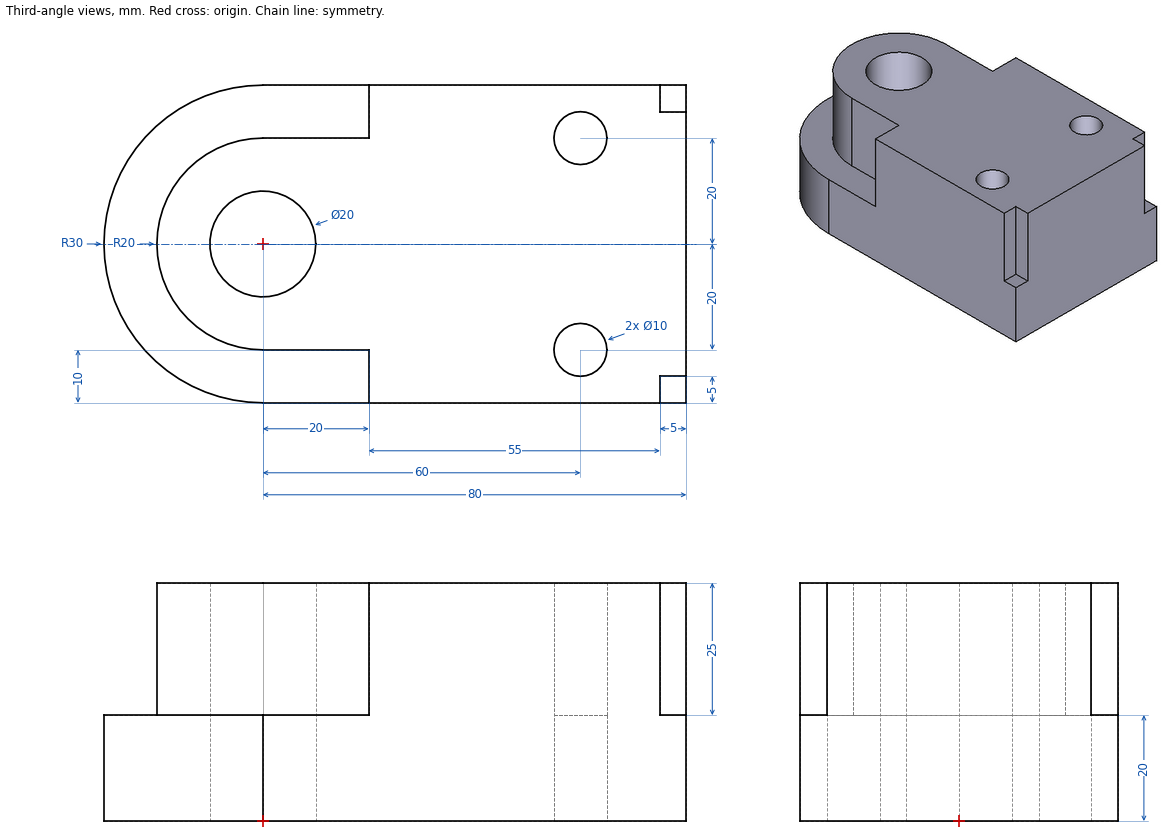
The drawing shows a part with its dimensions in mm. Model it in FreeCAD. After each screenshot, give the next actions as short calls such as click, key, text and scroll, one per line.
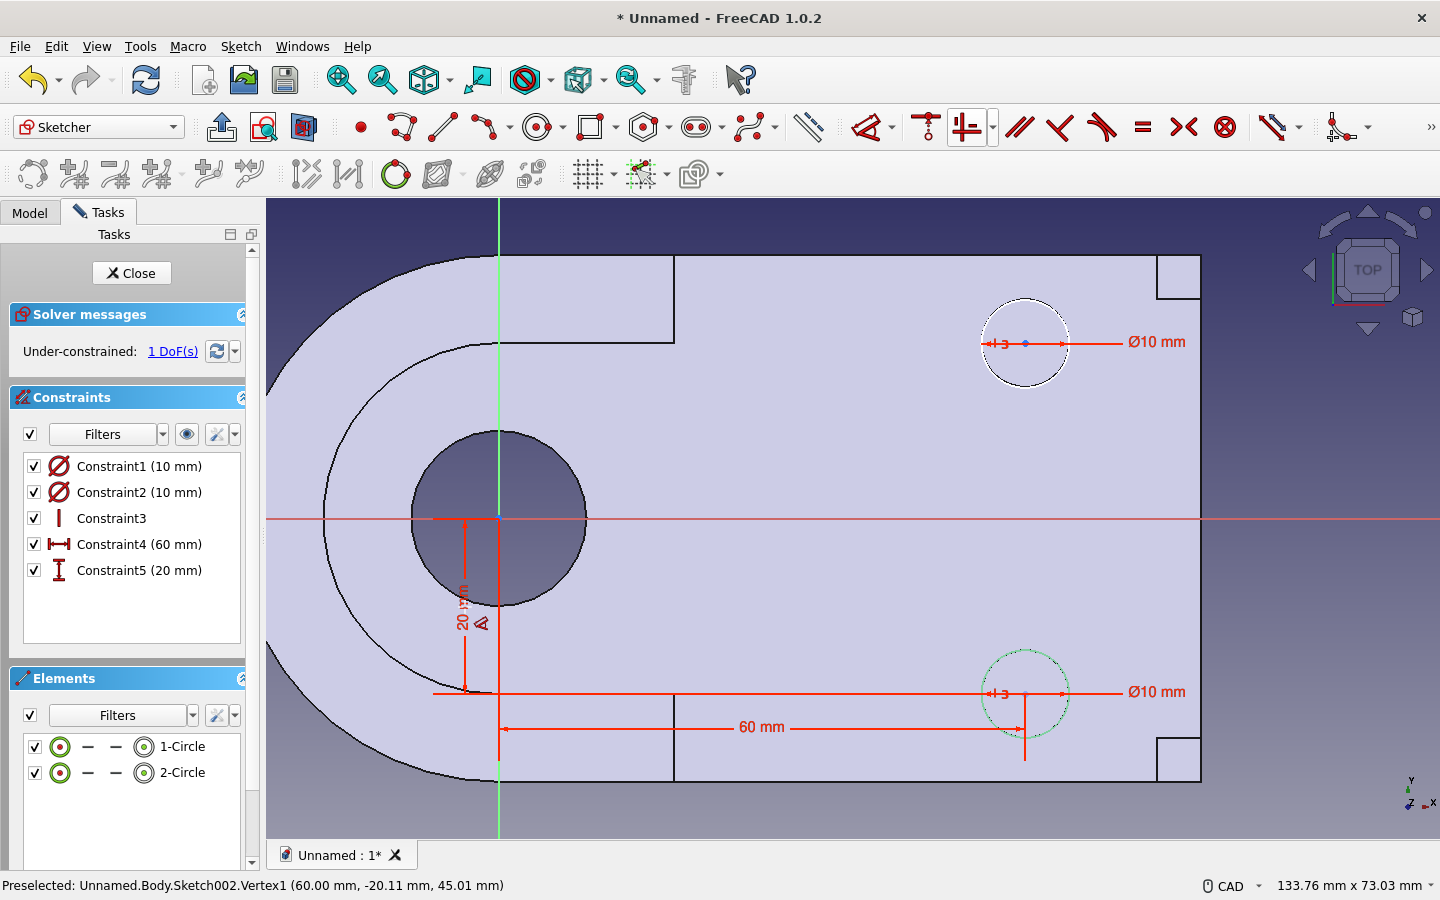
click(1025, 344)
click(465, 431)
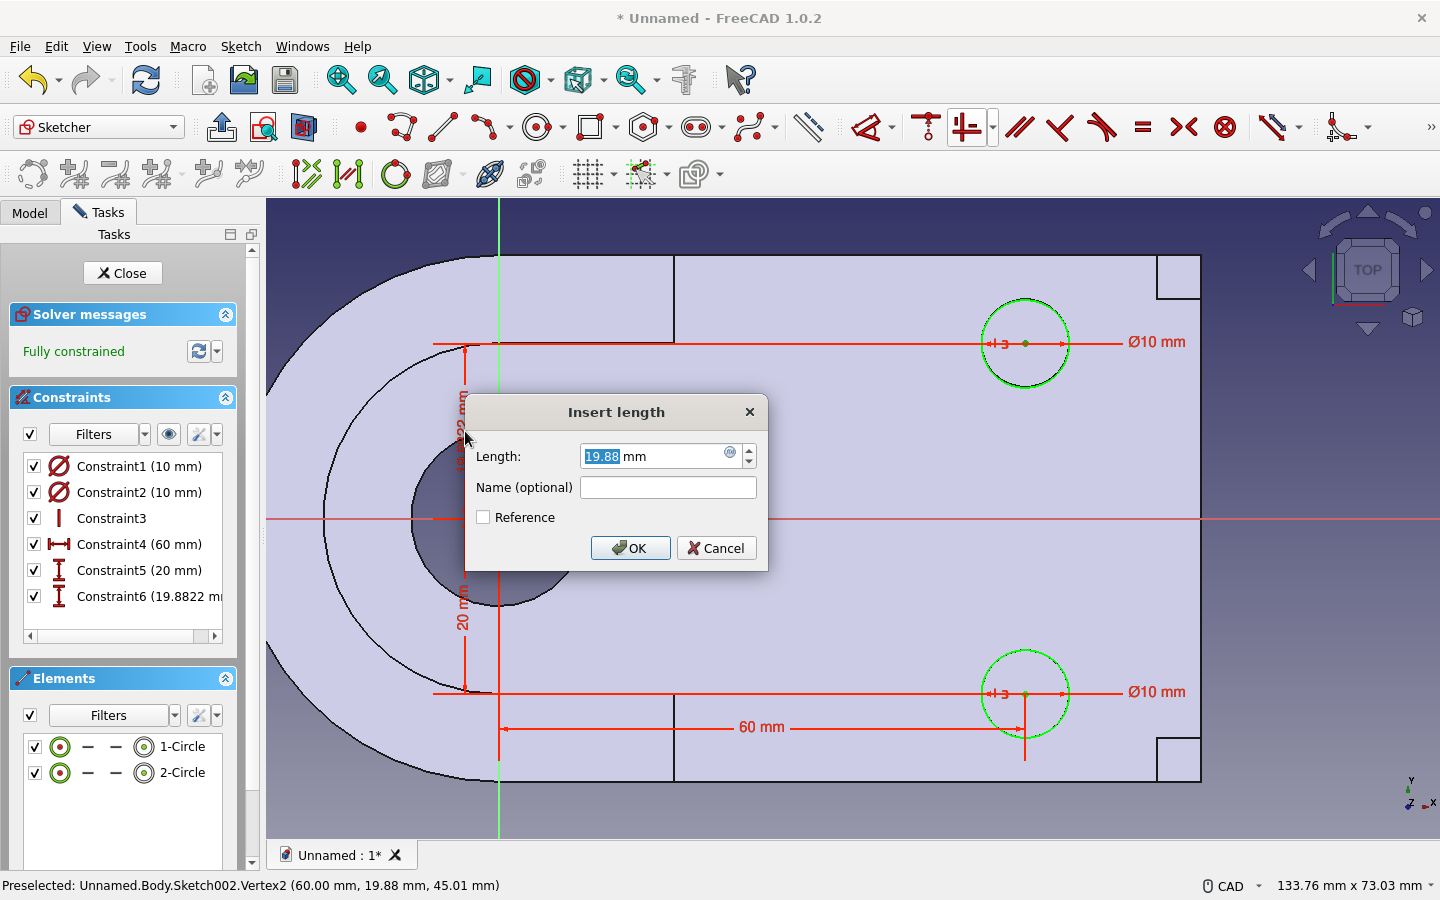
text(20)
key(Return)
key(Escape)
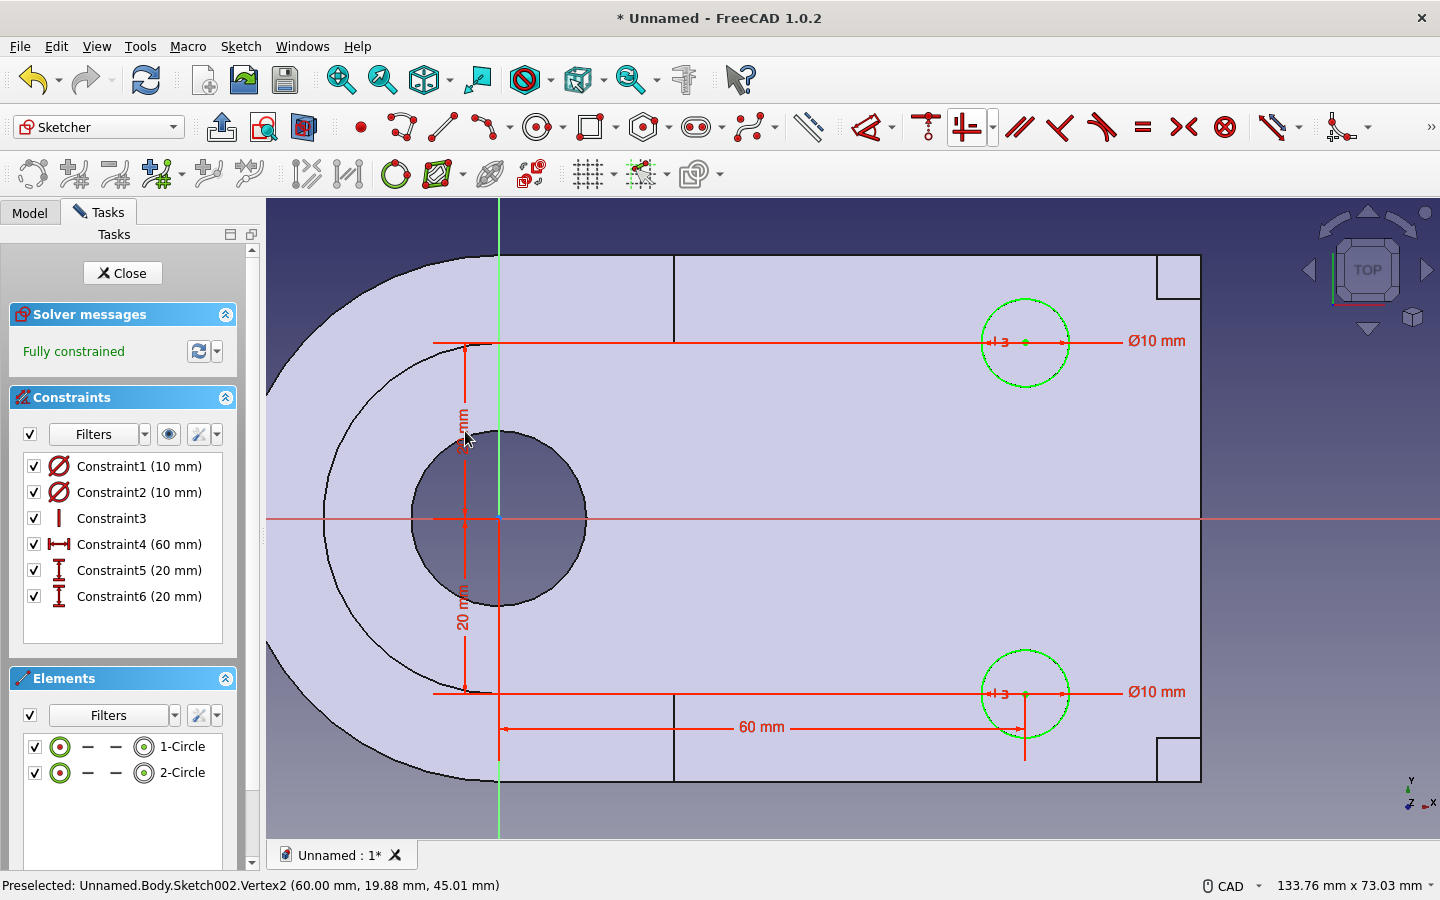
click(123, 273)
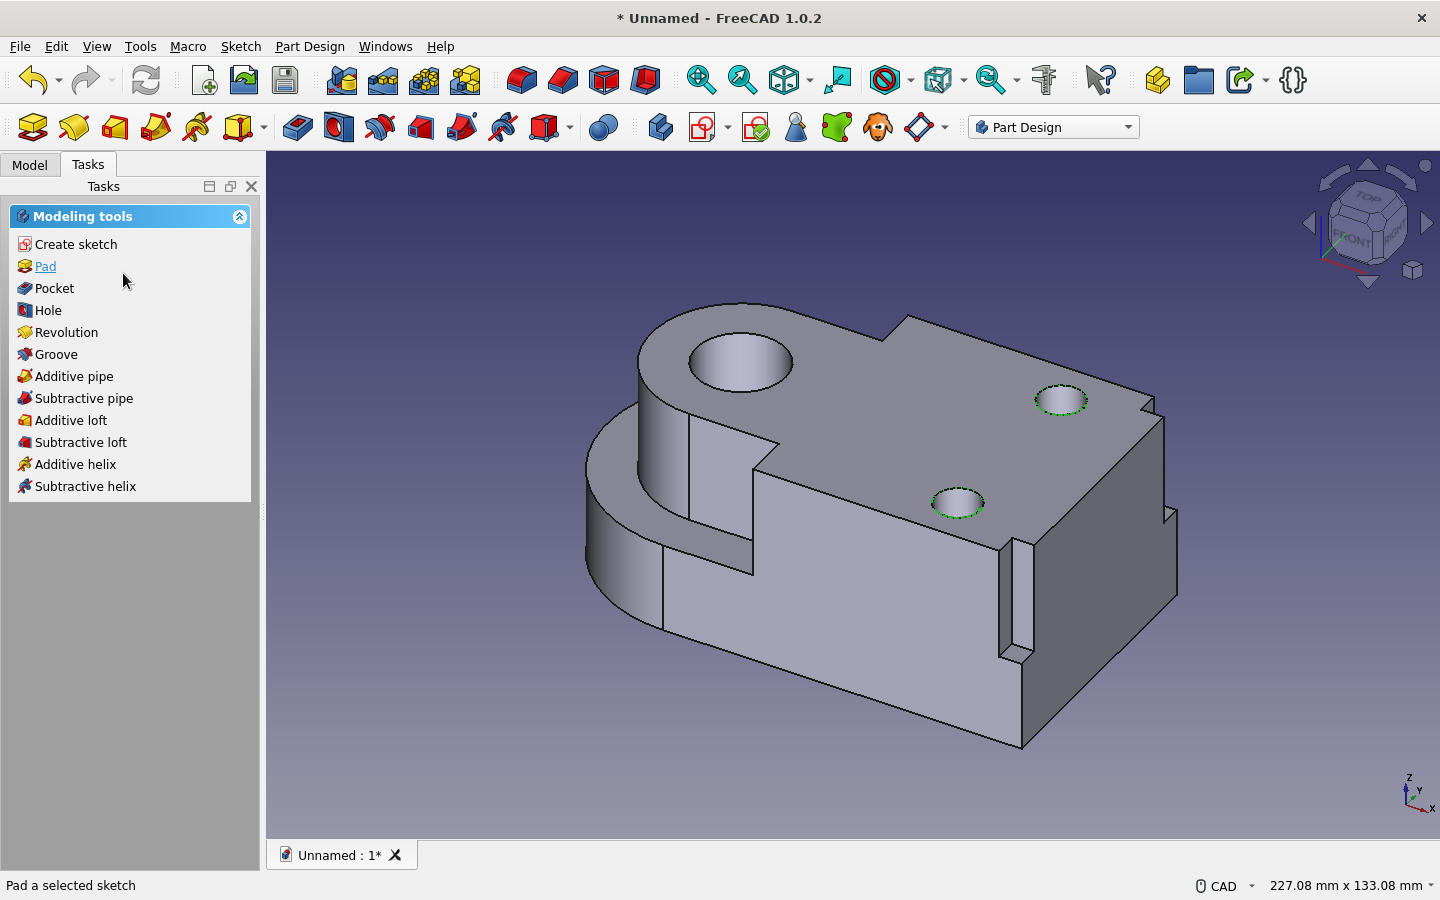
click(298, 128)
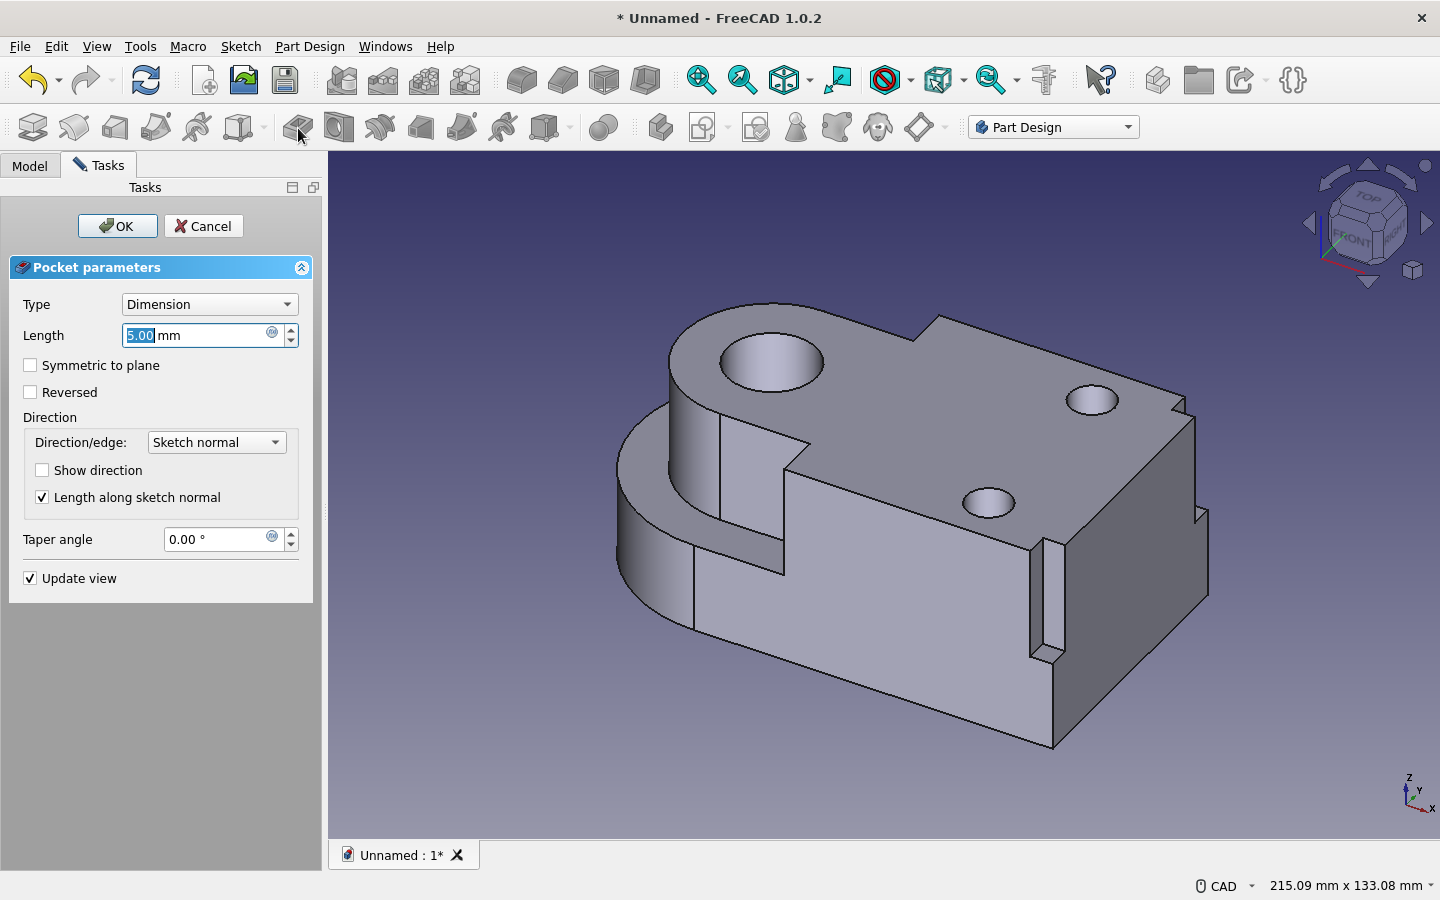
click(210, 304)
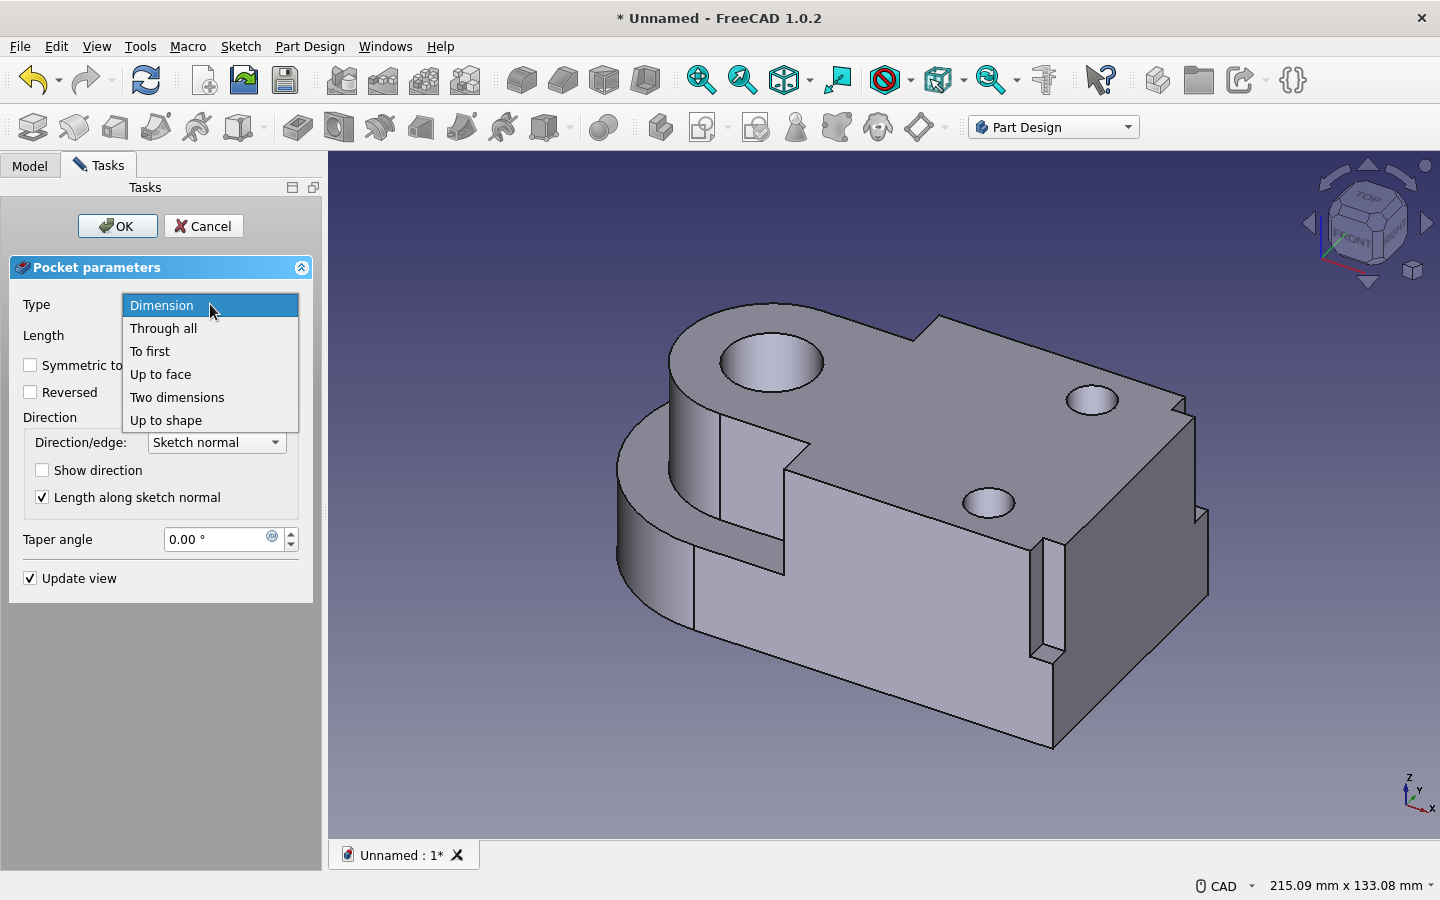
click(208, 328)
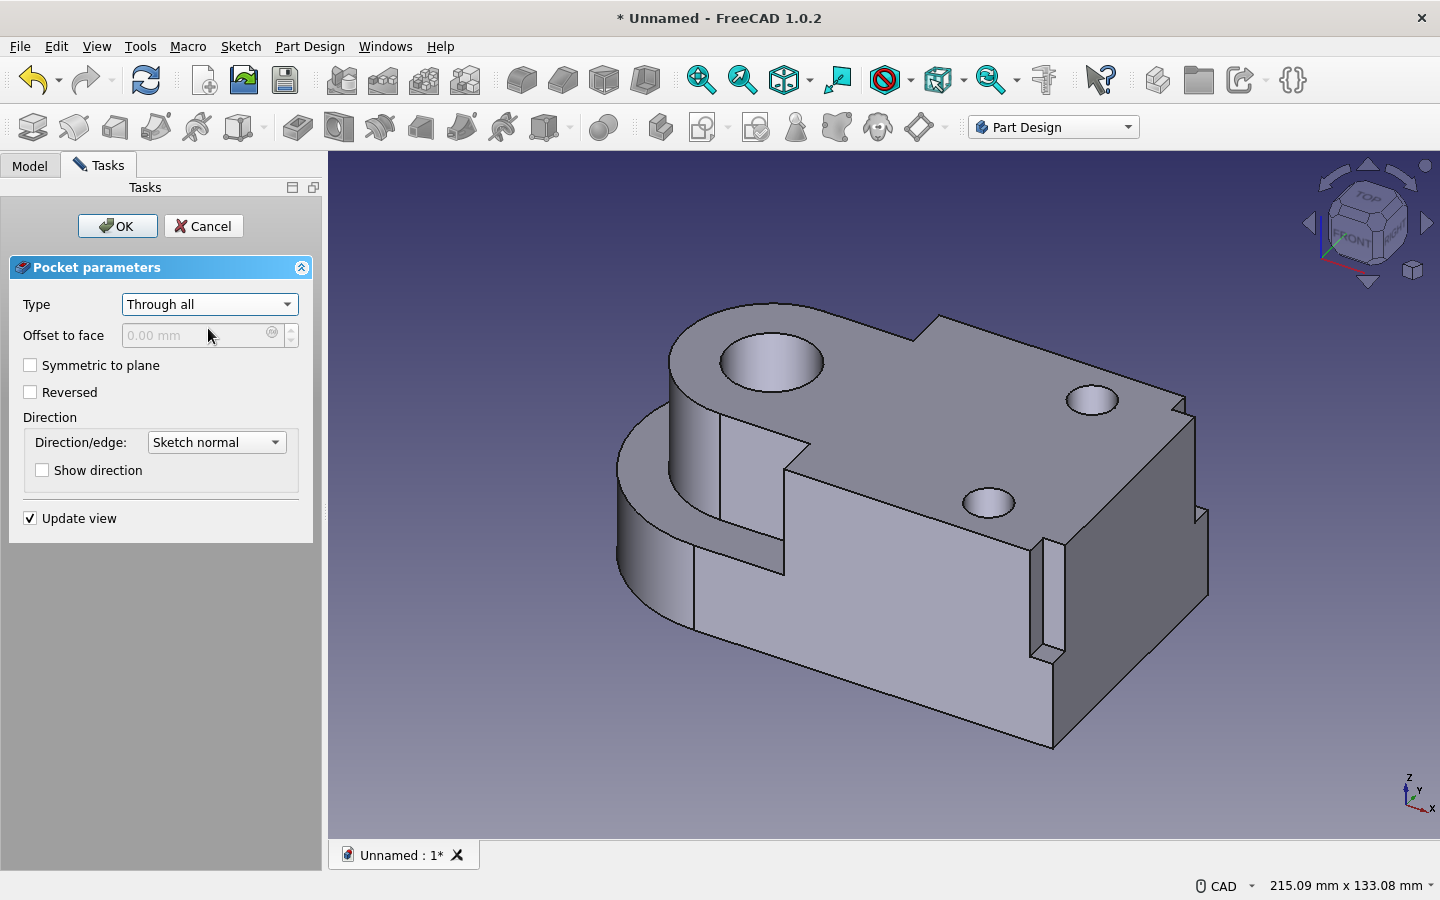
click(118, 226)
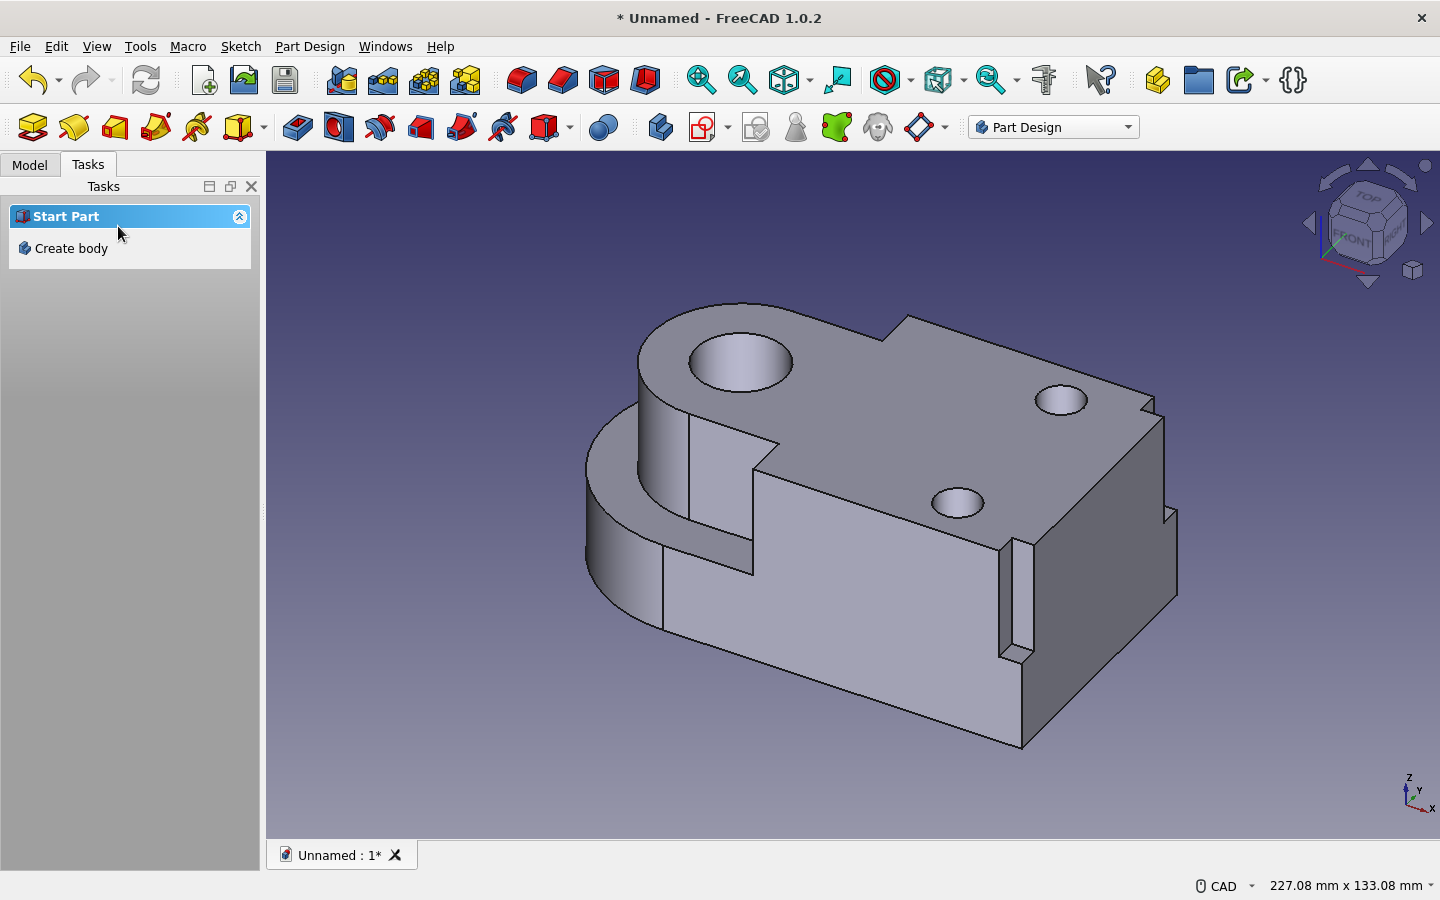
key(0)